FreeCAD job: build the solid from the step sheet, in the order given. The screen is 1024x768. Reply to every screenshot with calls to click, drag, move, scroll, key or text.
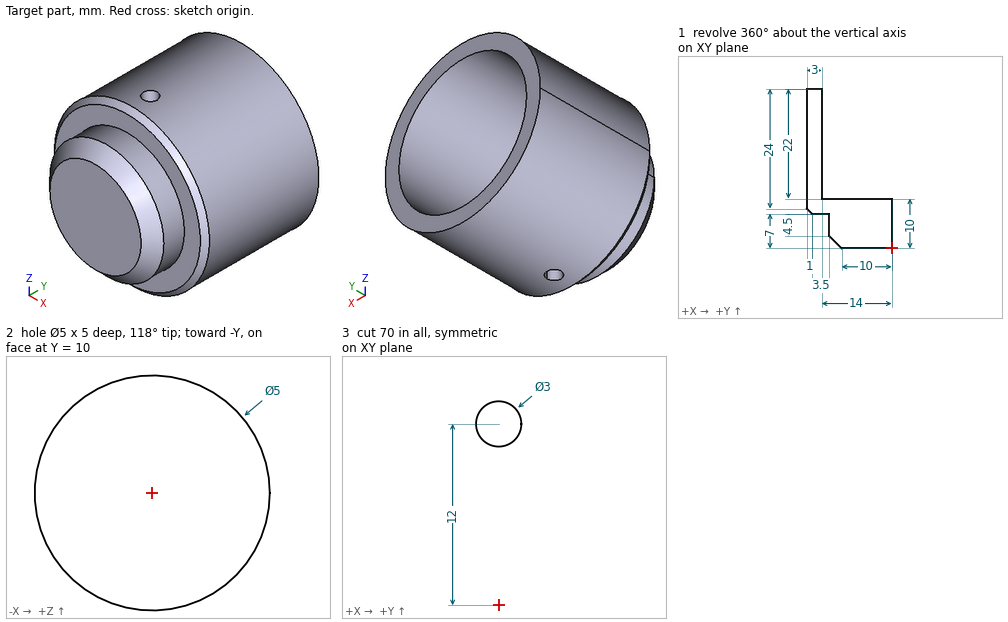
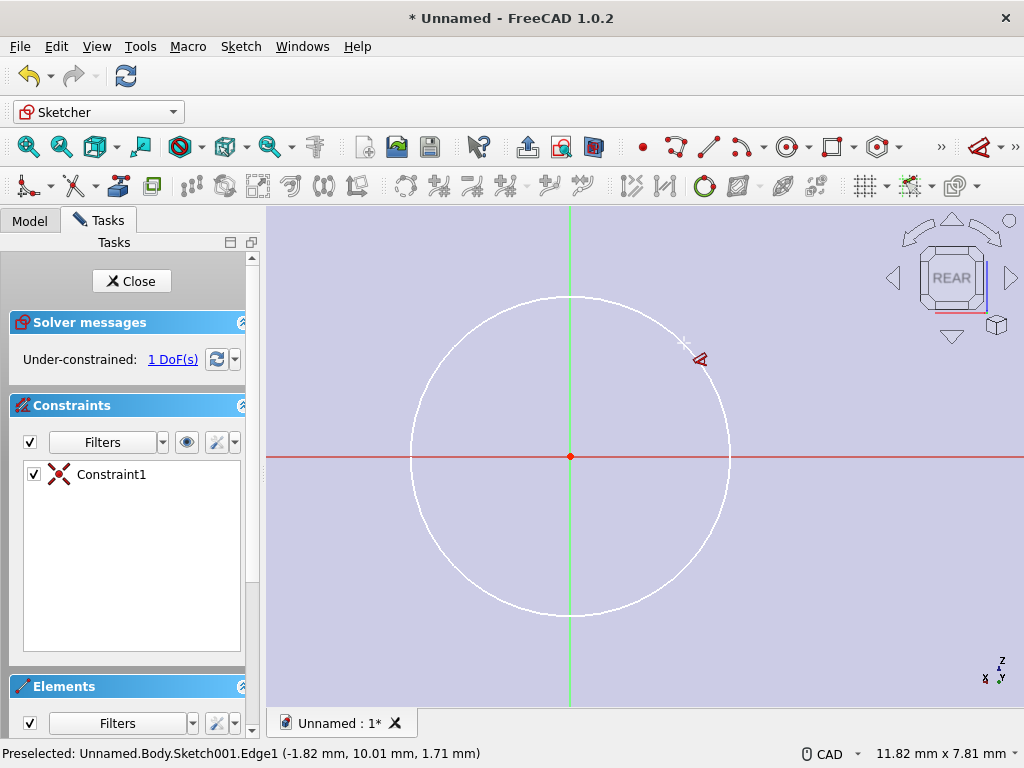
click(683, 343)
click(706, 320)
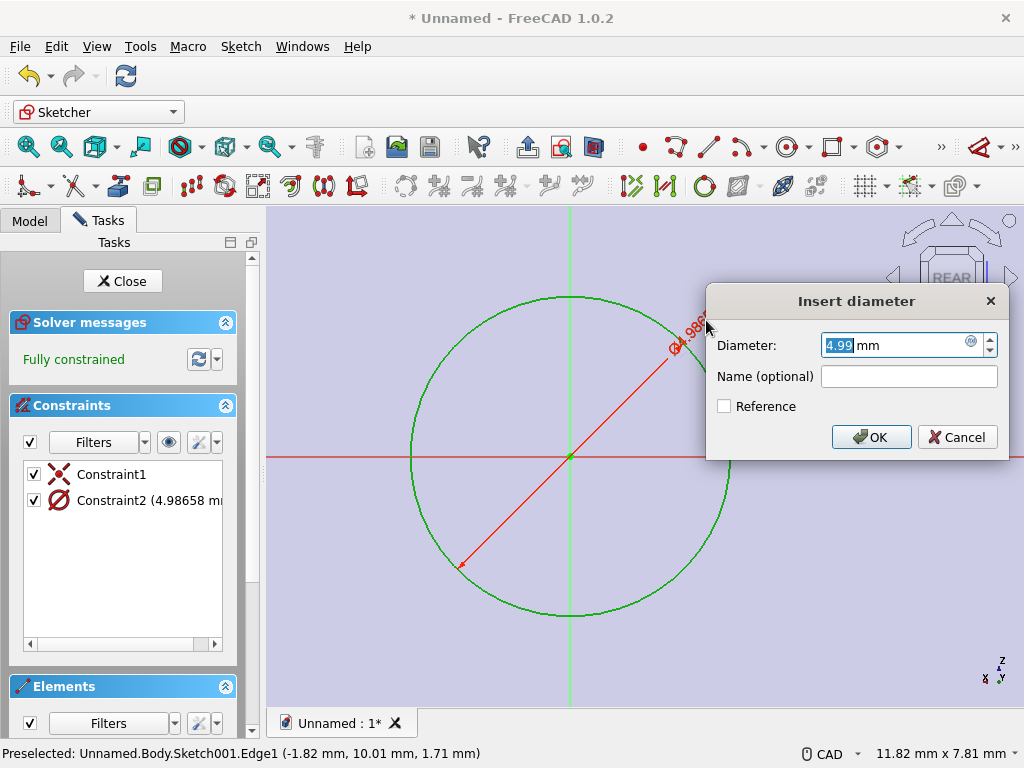
text(5)
key(Return)
key(Escape)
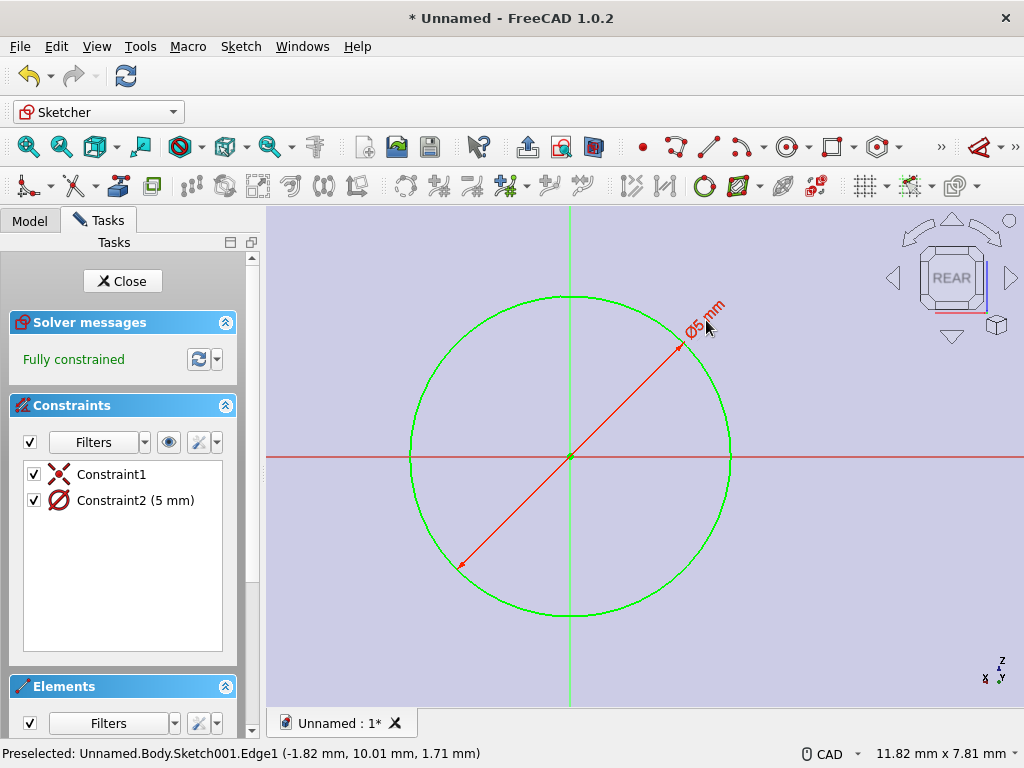
click(123, 281)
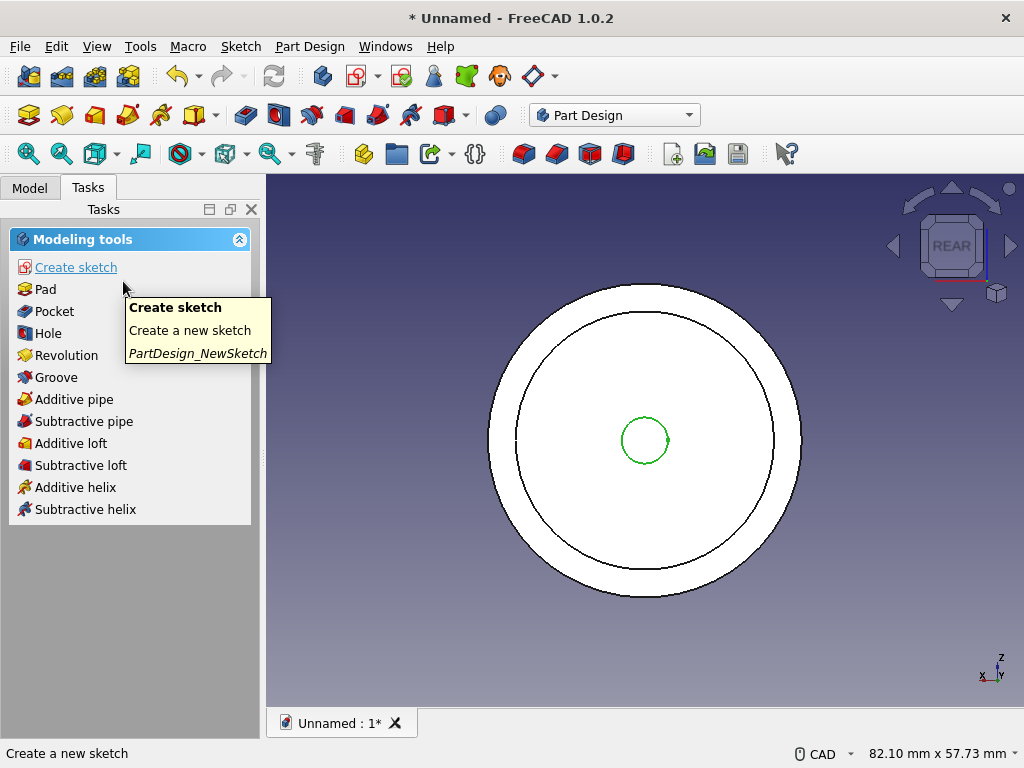
click(279, 116)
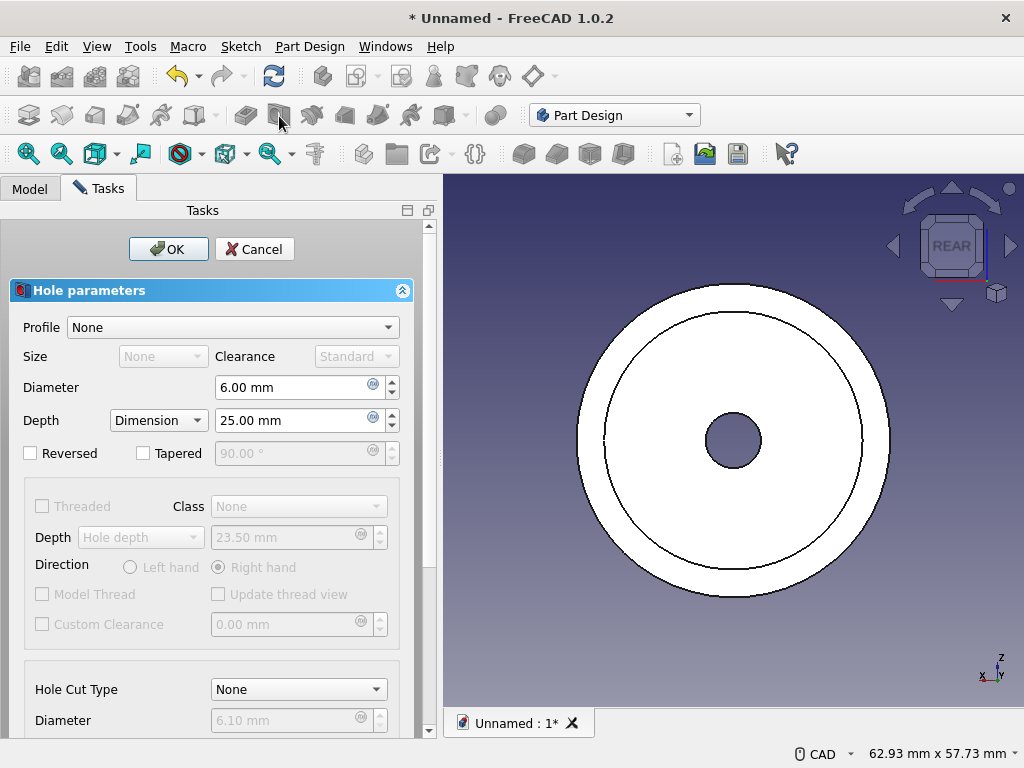
triple_click(300, 388)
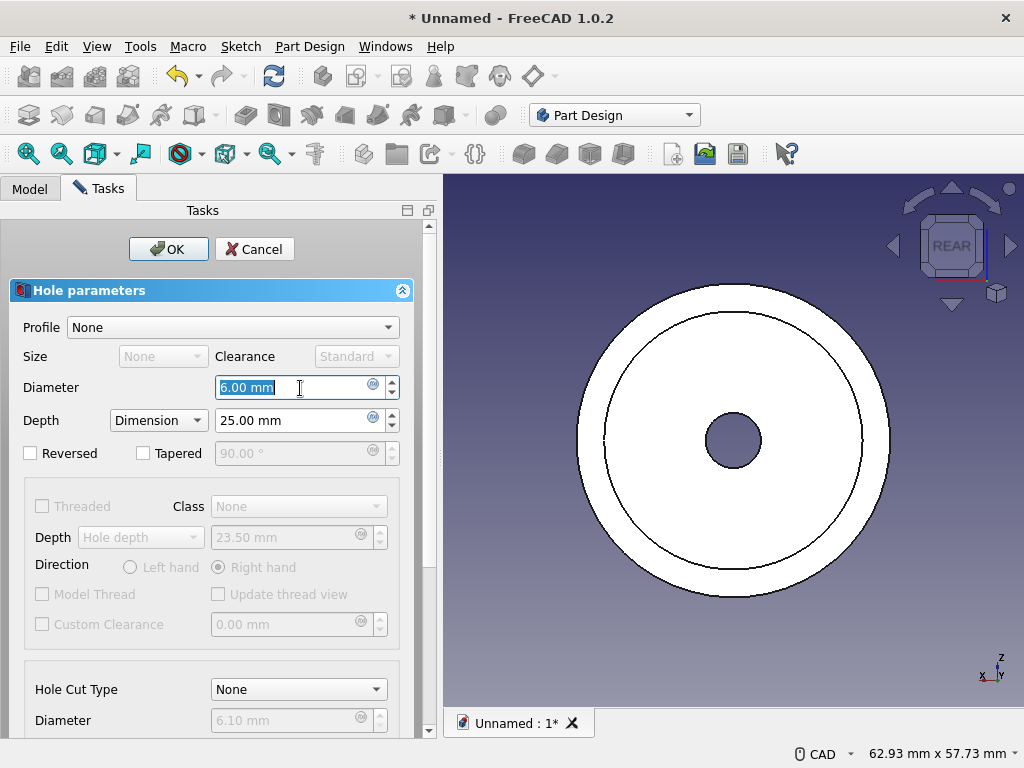
text(5)
key(Tab)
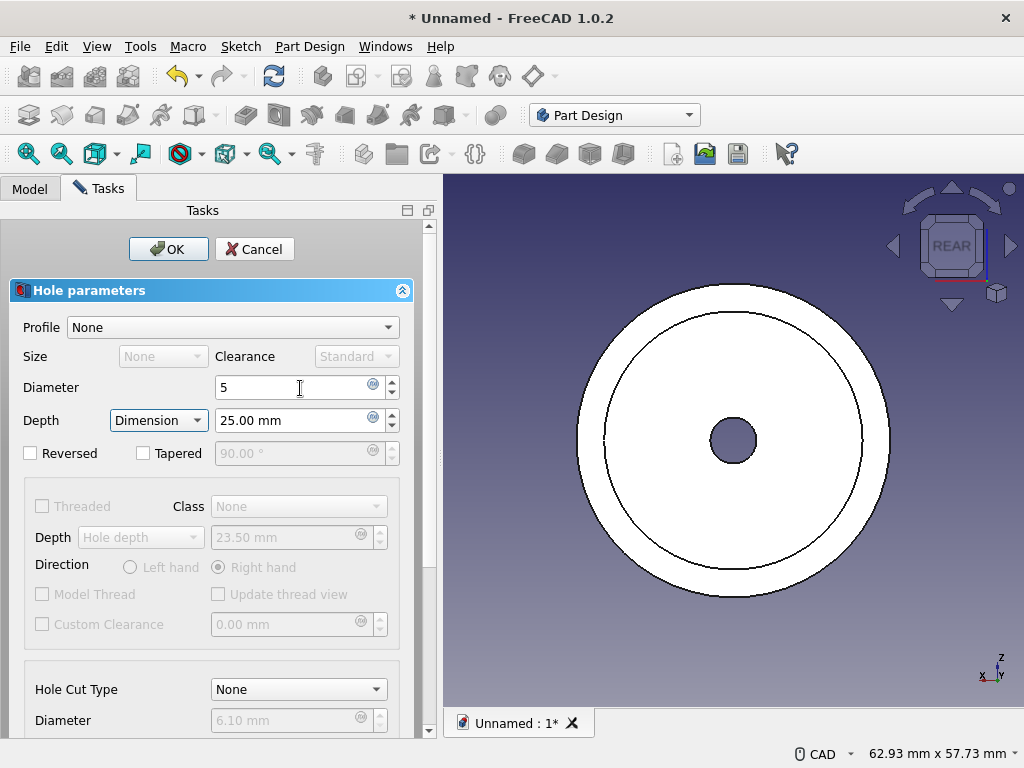
triple_click(300, 420)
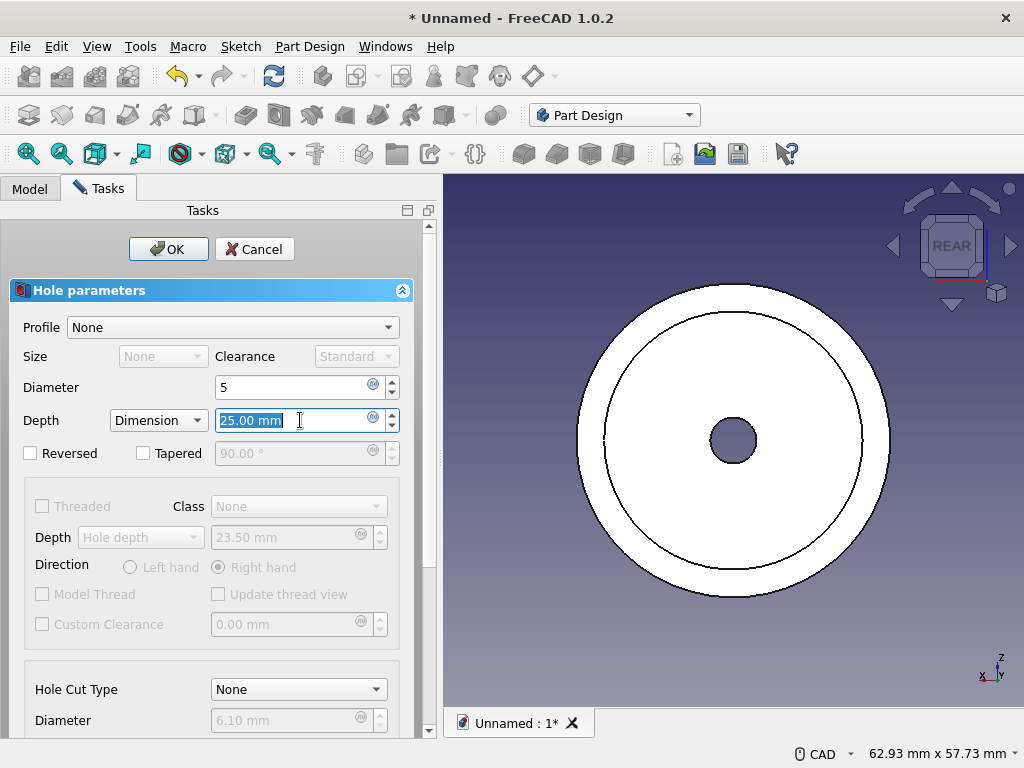
text(5)
key(Tab)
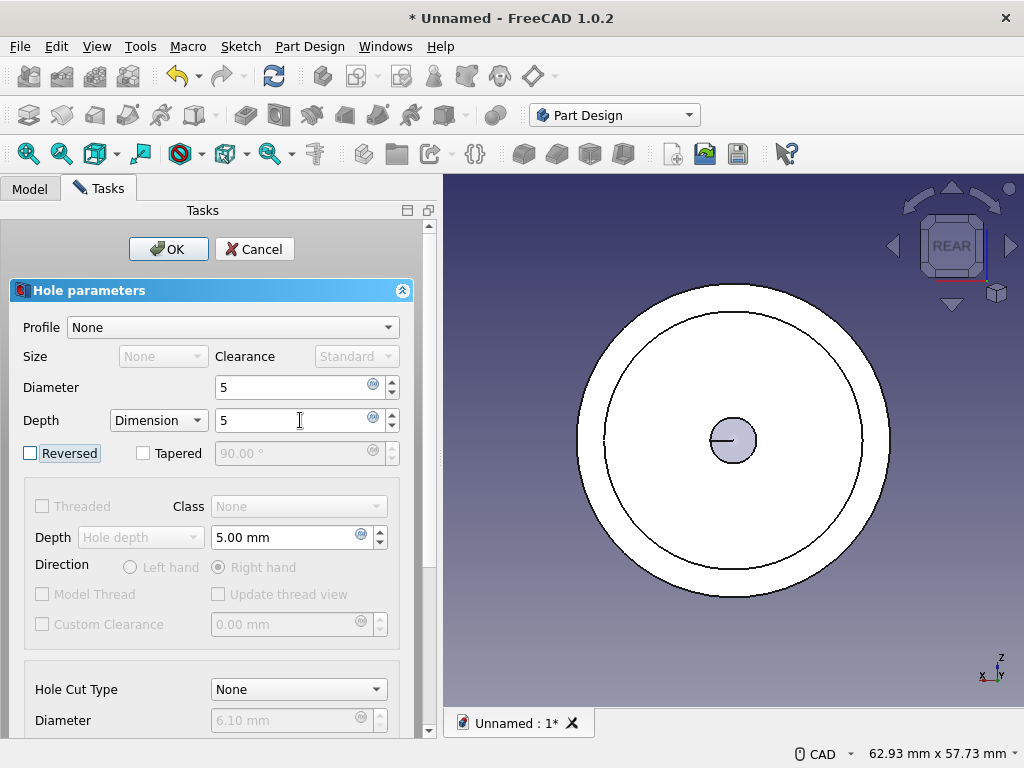
click(169, 249)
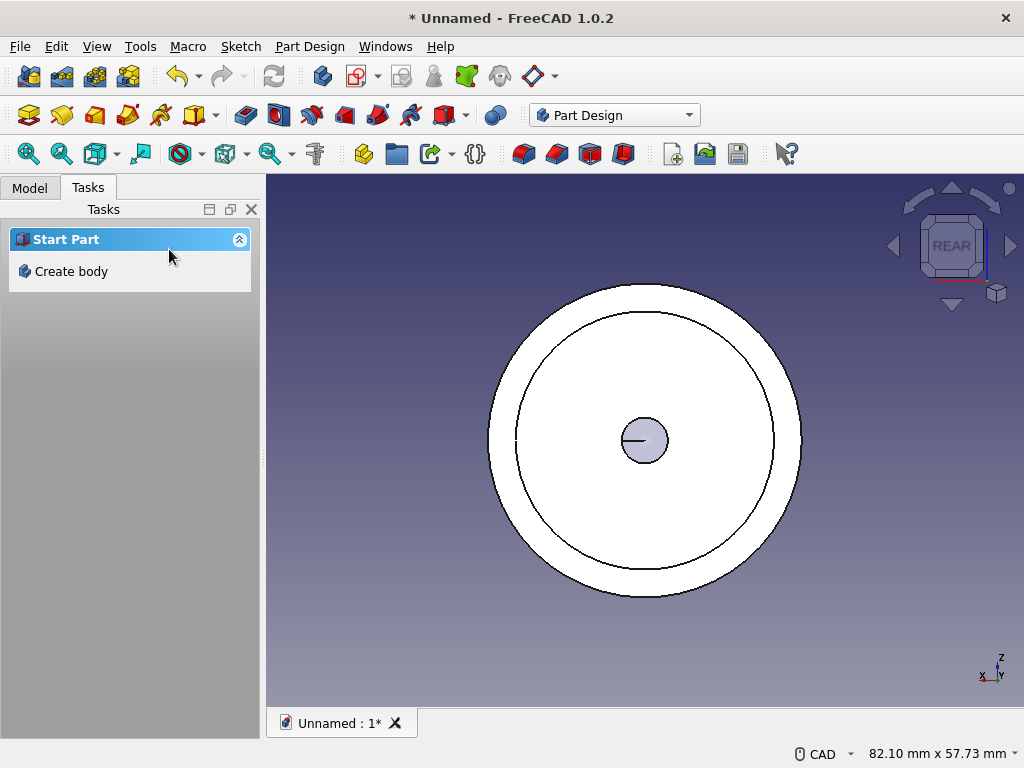
click(356, 76)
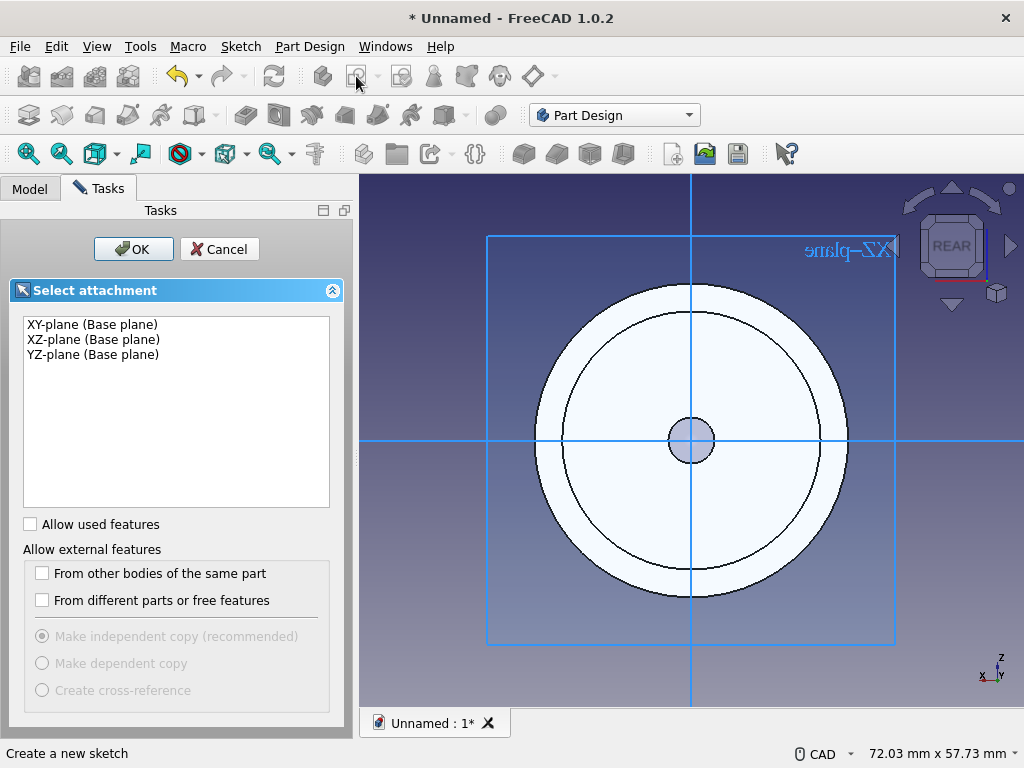
click(84, 324)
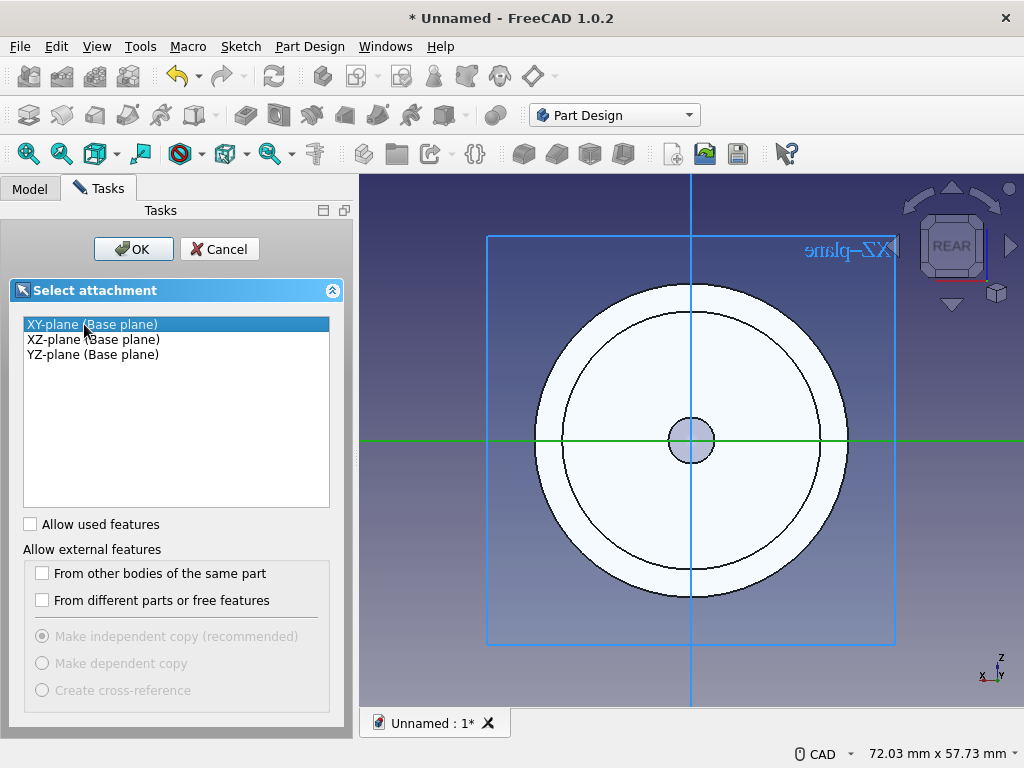
click(134, 249)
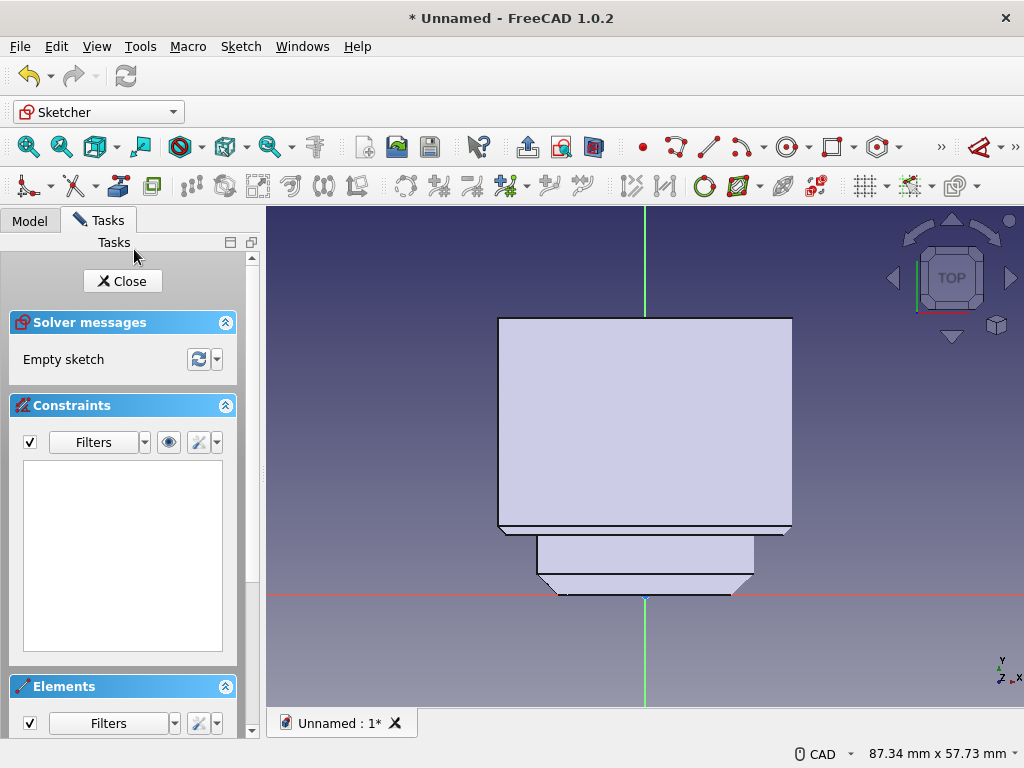
key(q)
key(s)